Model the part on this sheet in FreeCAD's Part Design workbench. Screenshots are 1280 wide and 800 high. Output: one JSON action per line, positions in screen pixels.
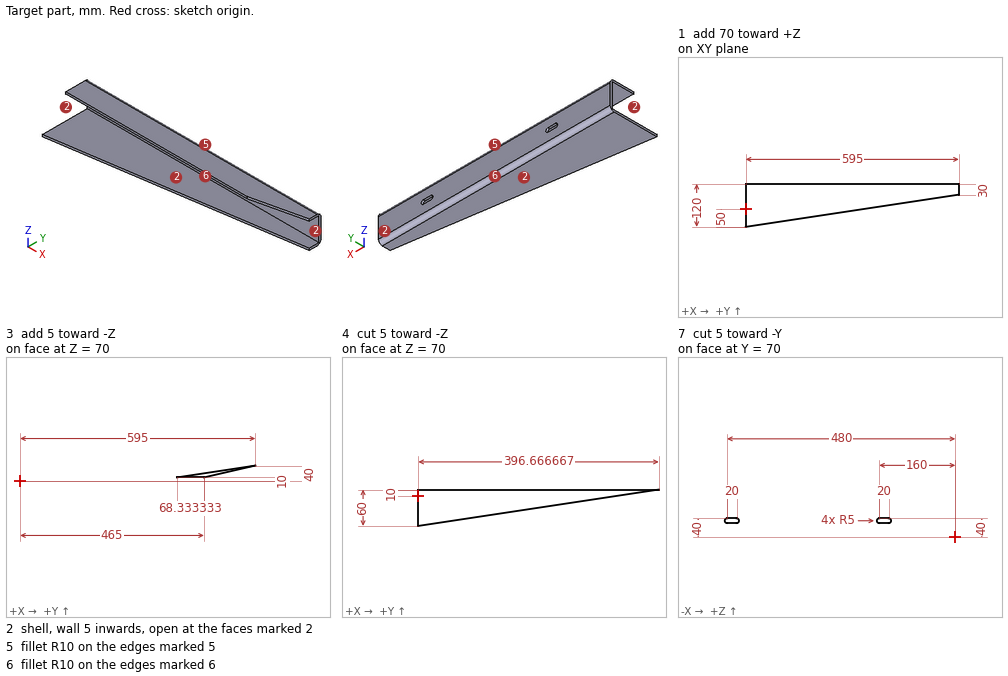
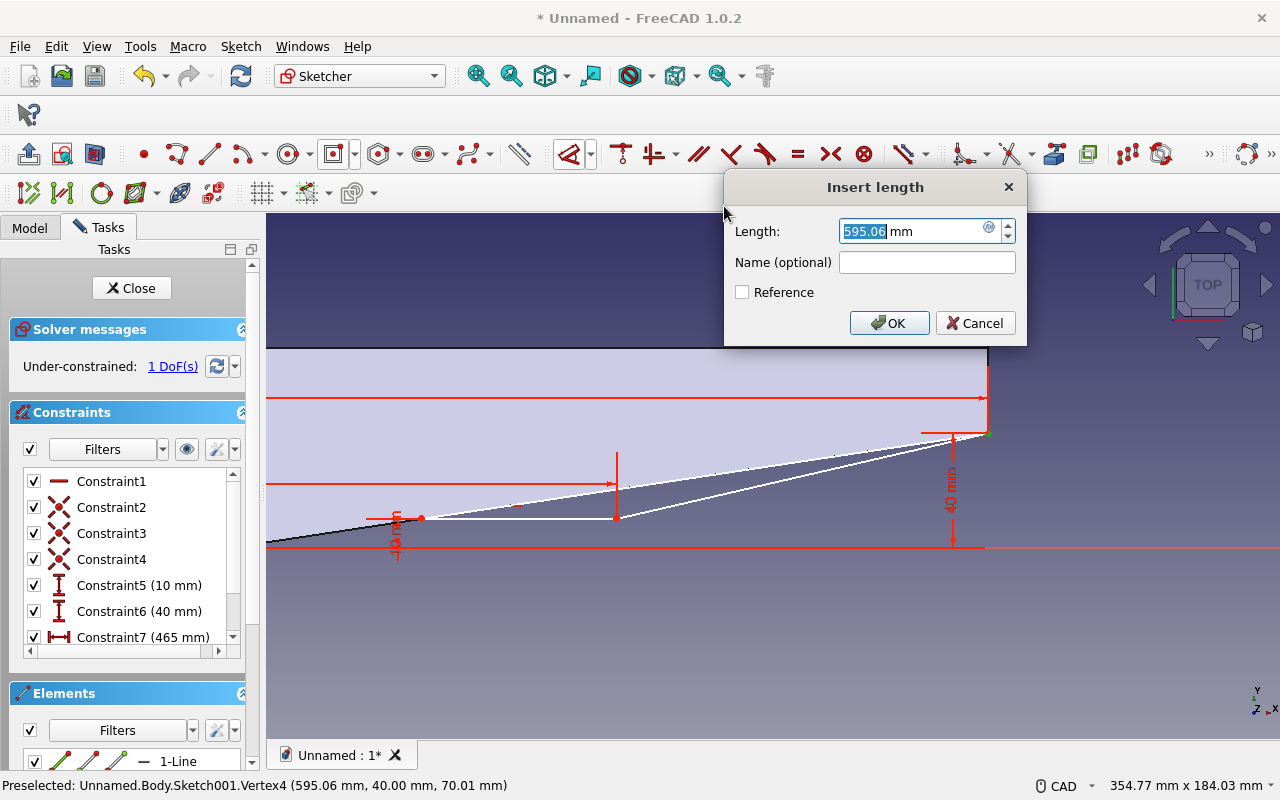
{"action": "type", "text": "595"}
{"action": "key", "text": "Return"}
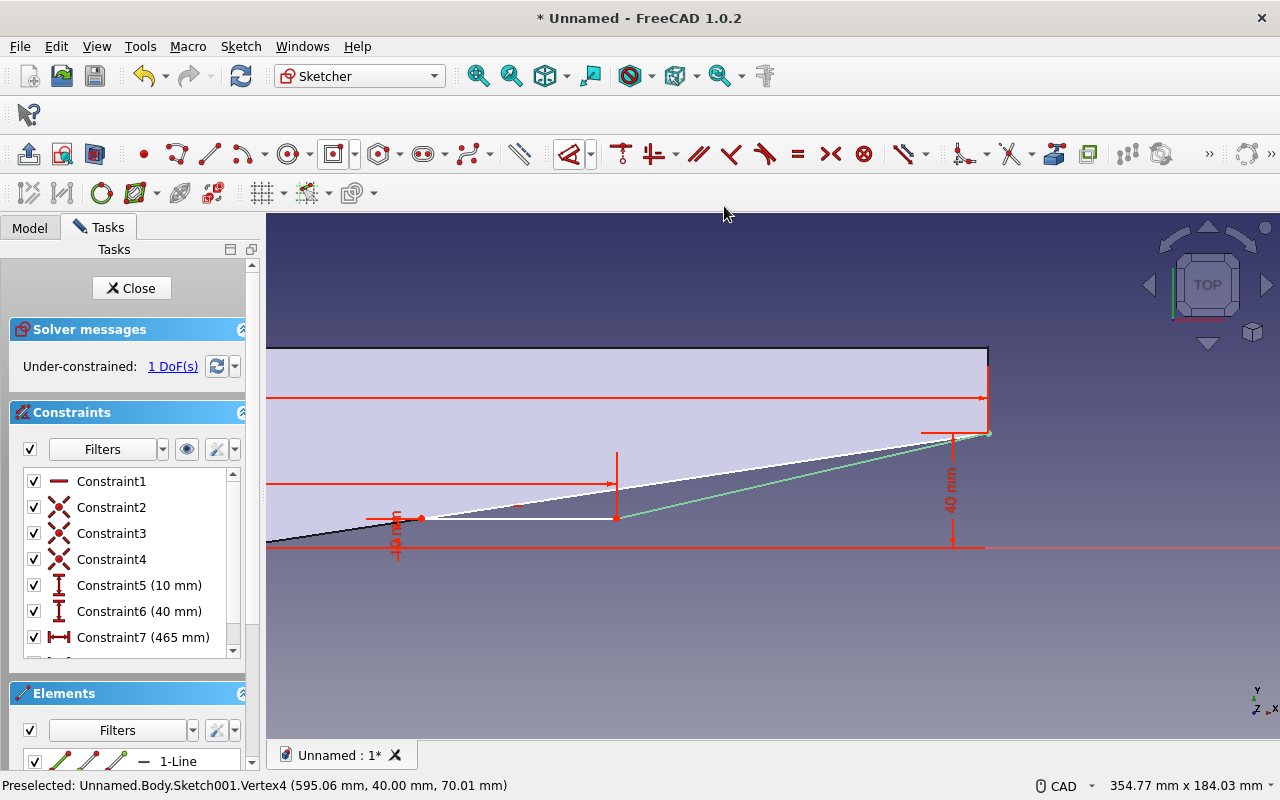
{"action": "left_click", "coordinate": [558, 519]}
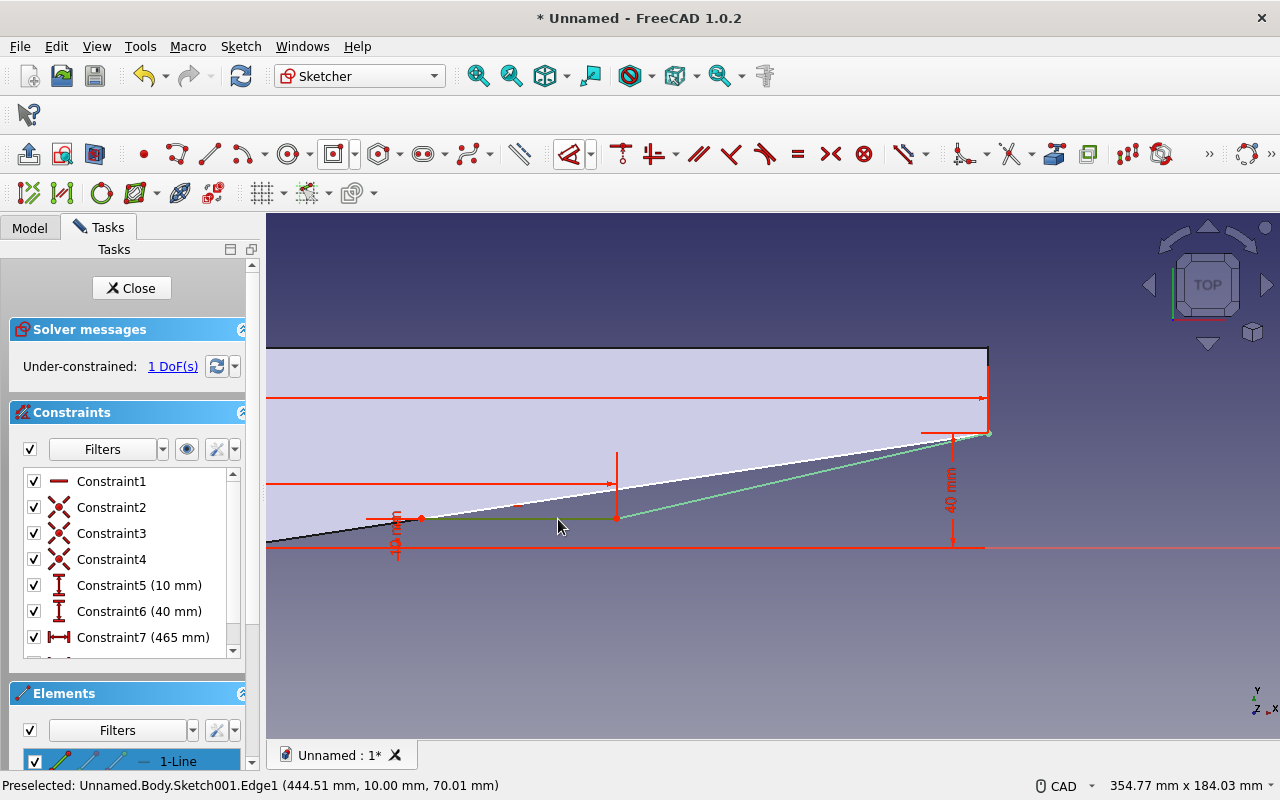
{"action": "left_click", "coordinate": [590, 154]}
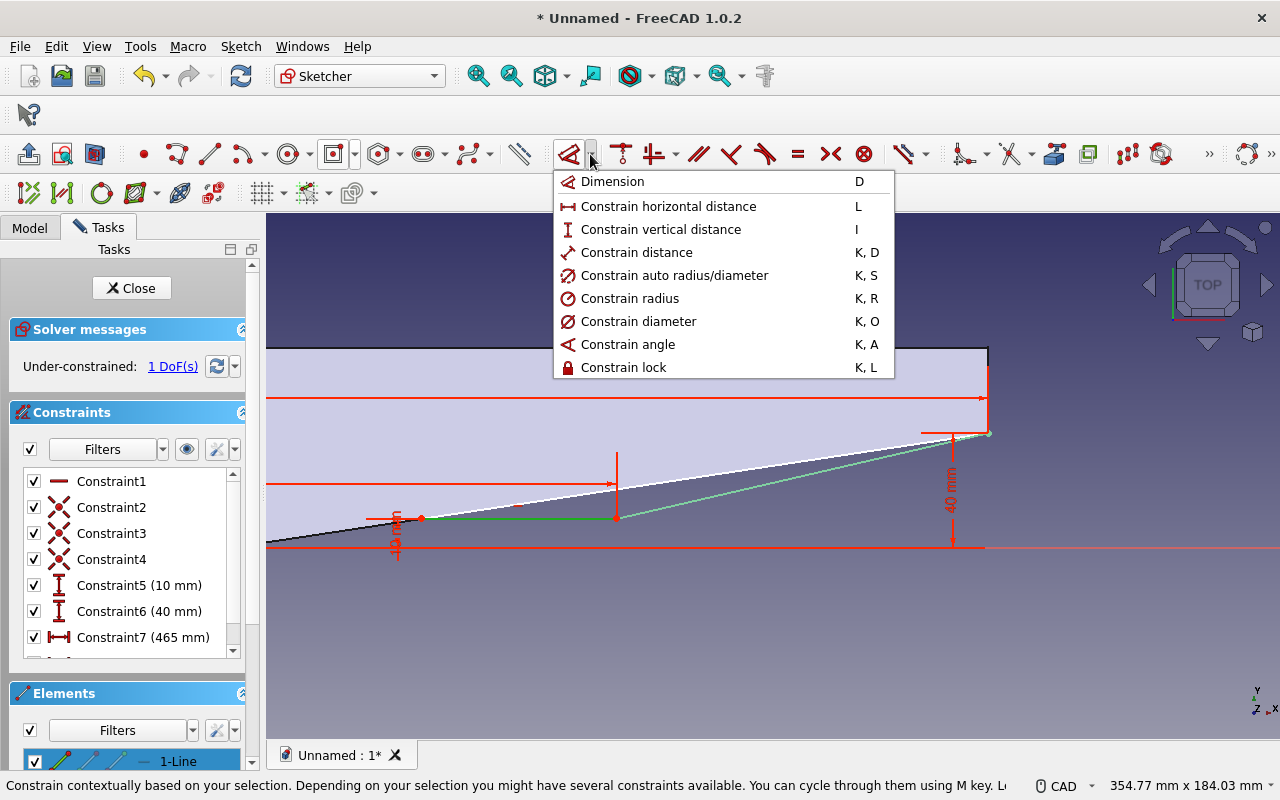
{"action": "left_click", "coordinate": [724, 206]}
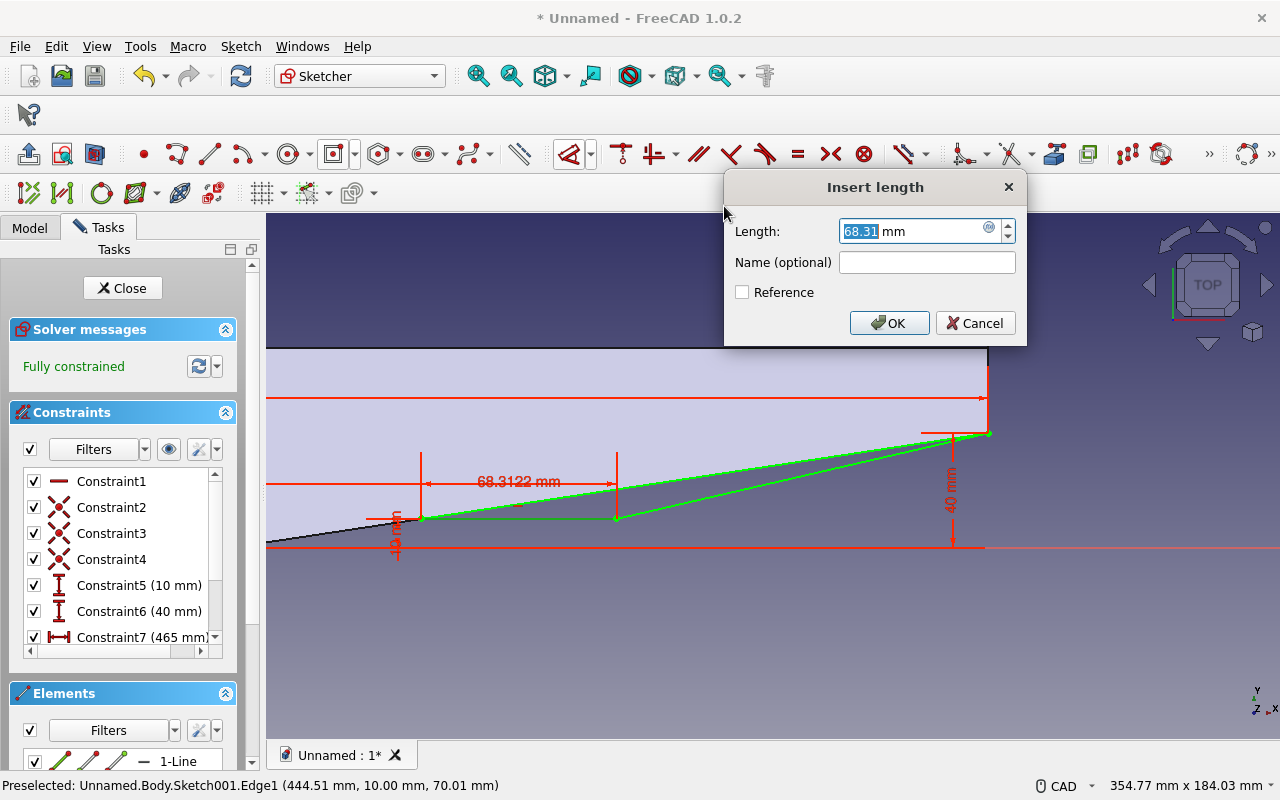
{"action": "type", "text": "68.333333"}
{"action": "key", "text": "Return"}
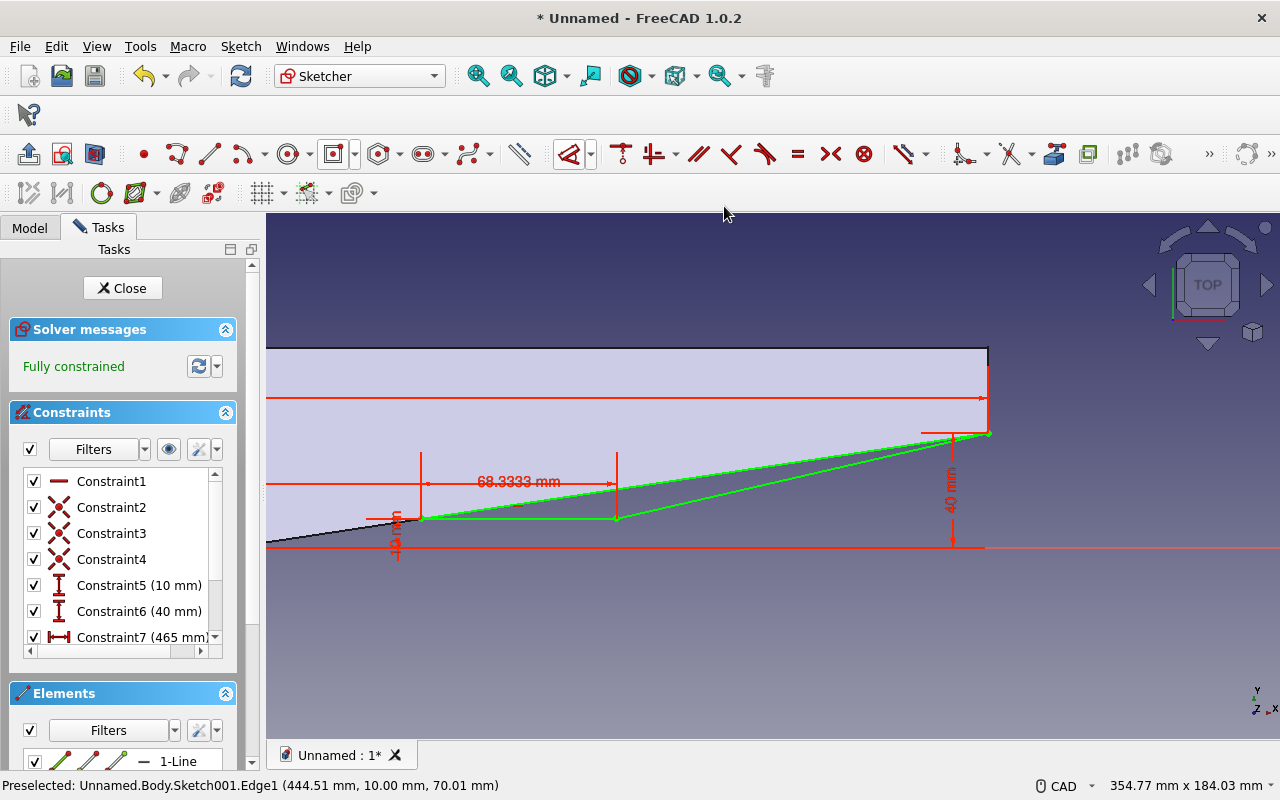
{"action": "left_click", "coordinate": [123, 288]}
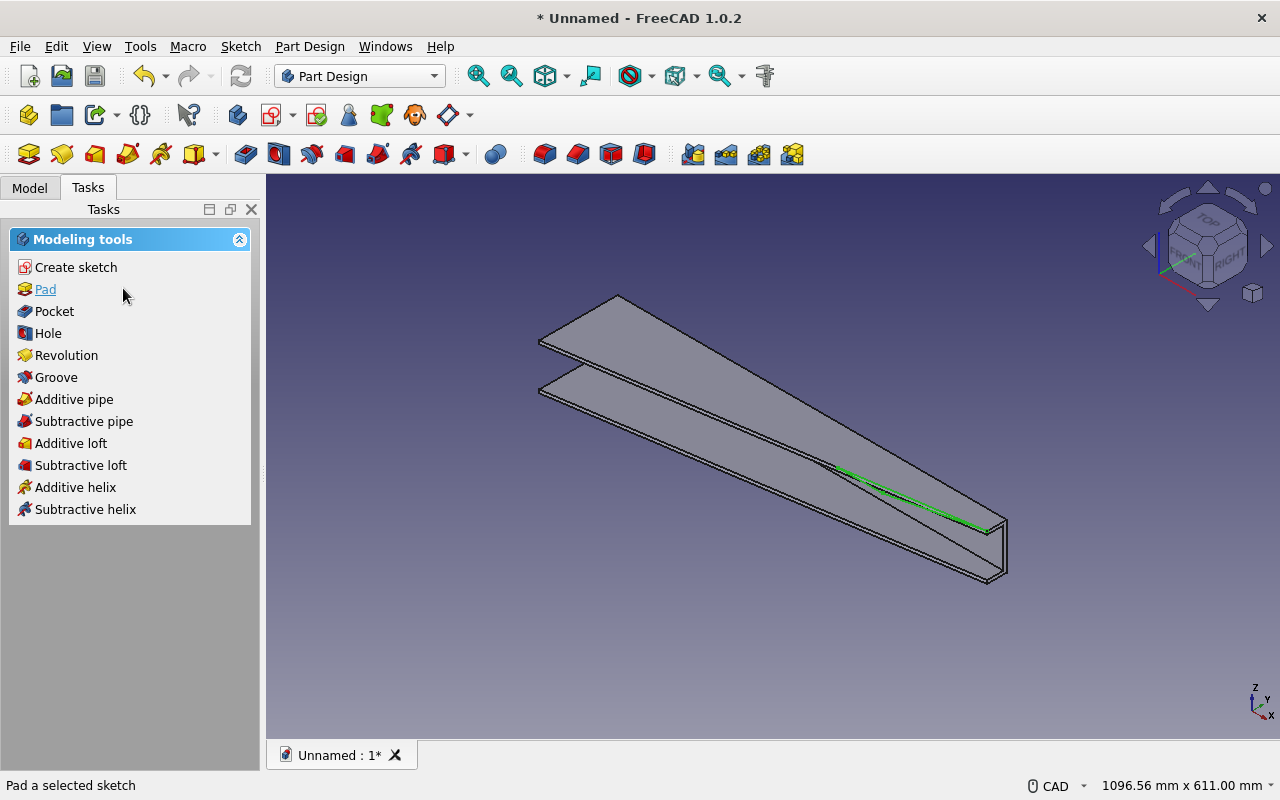
{"action": "left_click", "coordinate": [29, 154]}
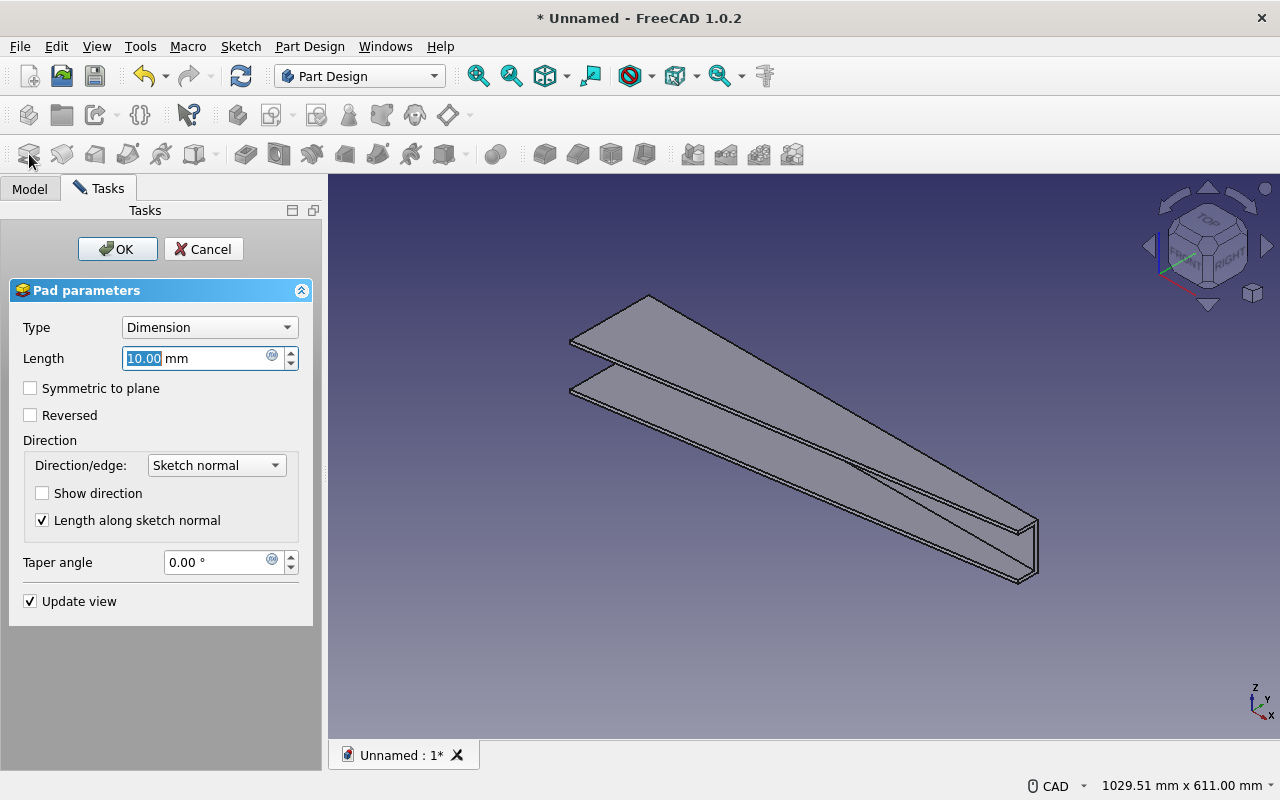
{"action": "type", "text": "5"}
{"action": "key", "text": "Tab"}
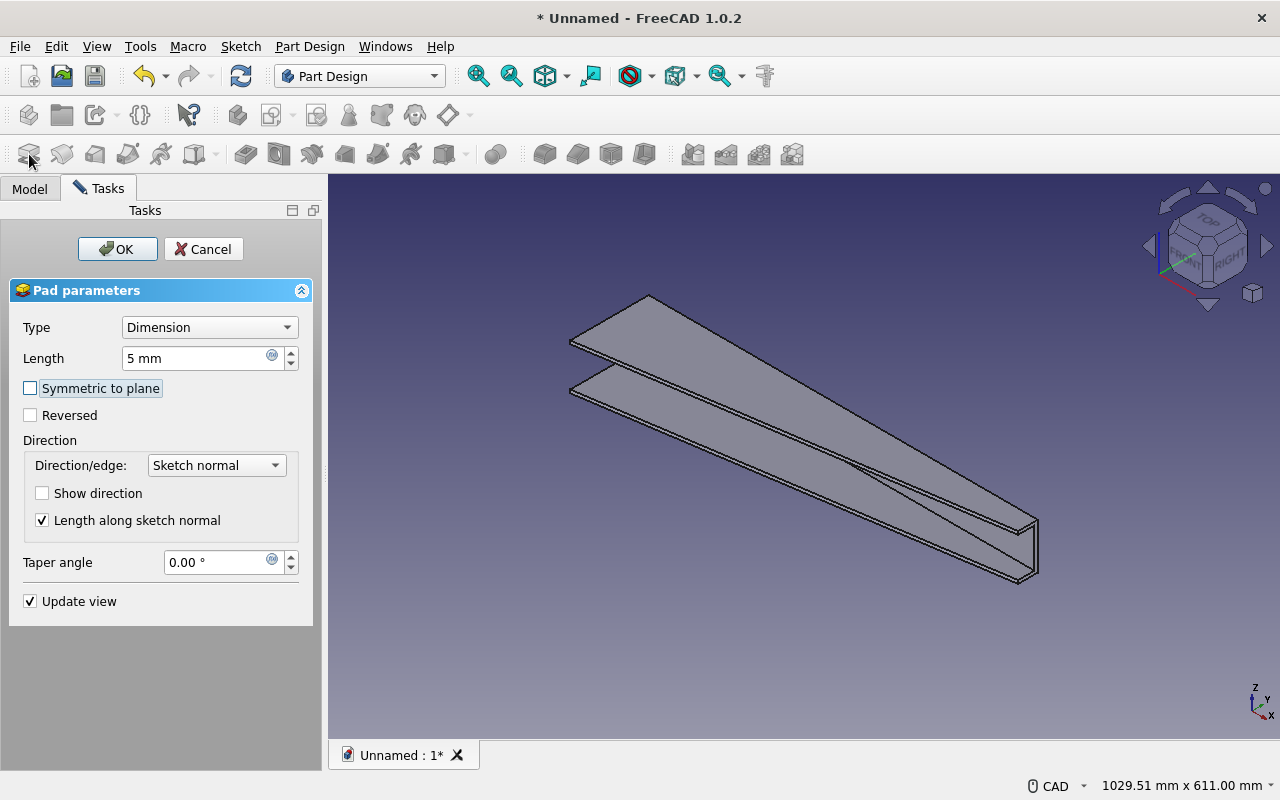
{"action": "left_click", "coordinate": [31, 415]}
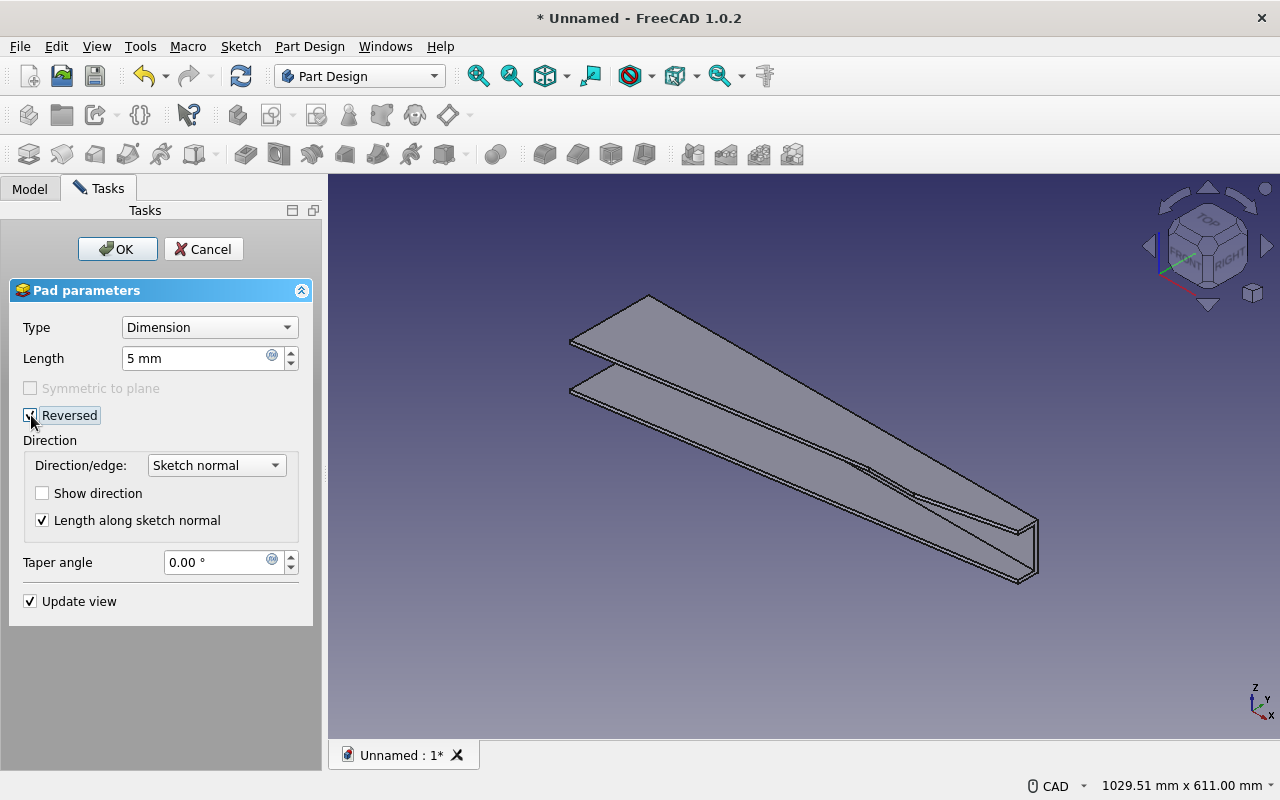
{"action": "left_click", "coordinate": [118, 249]}